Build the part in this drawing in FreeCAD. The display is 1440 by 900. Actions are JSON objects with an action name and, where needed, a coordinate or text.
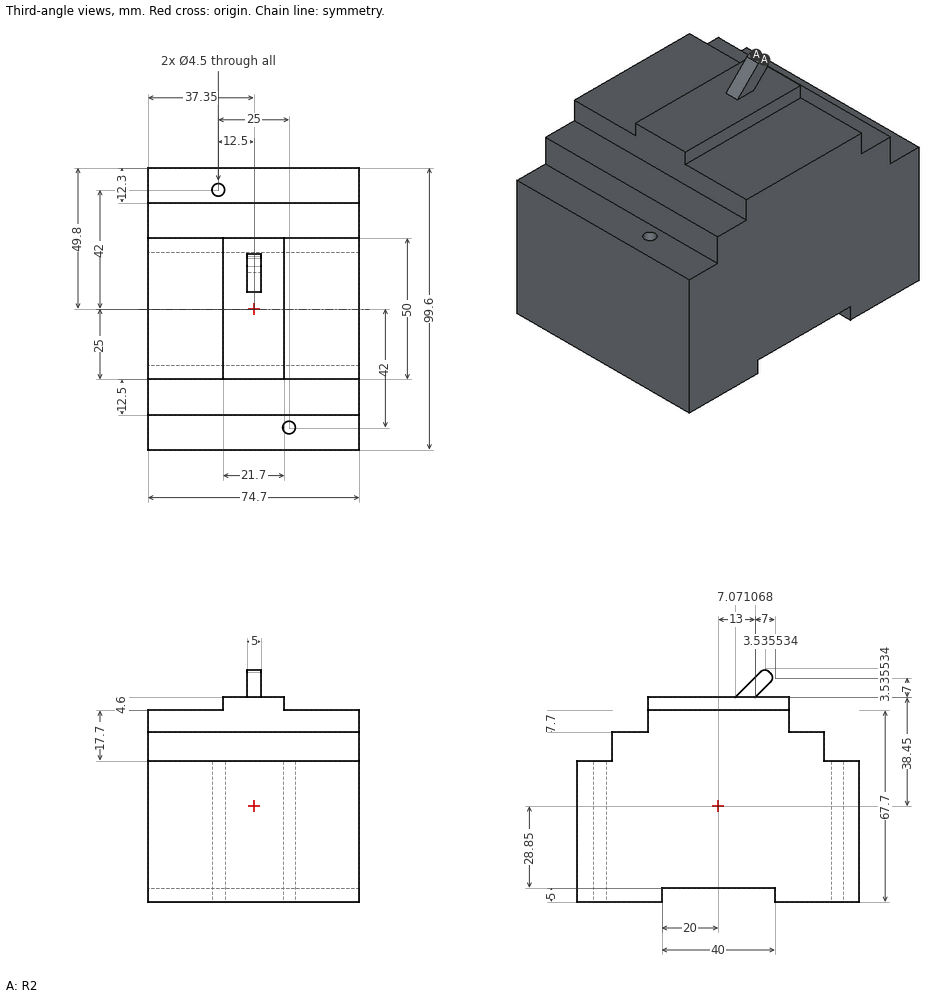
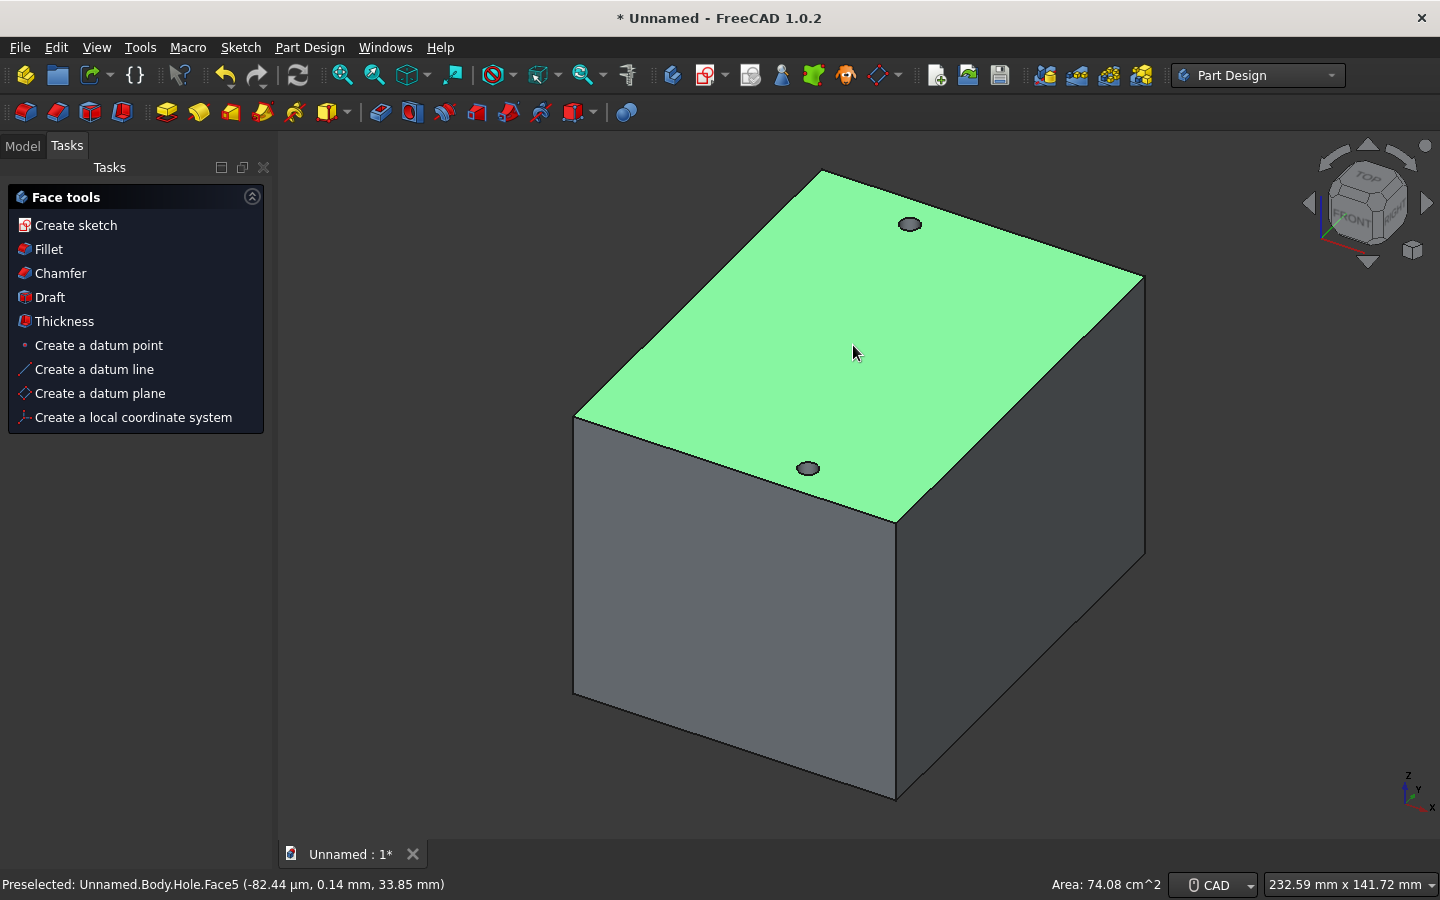
{"action": "left_click", "coordinate": [706, 76]}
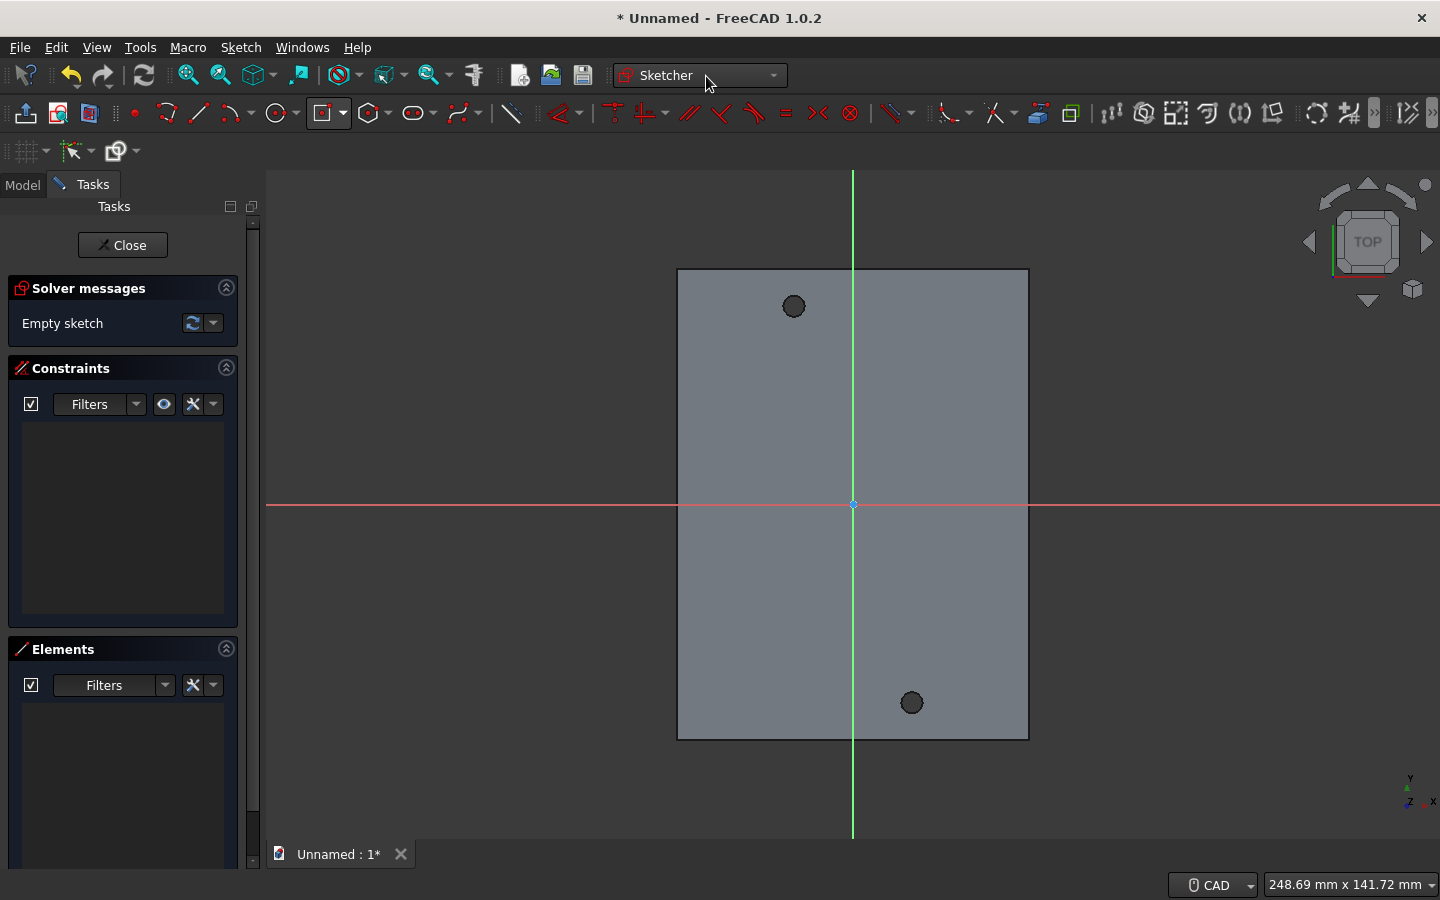
{"action": "left_click", "coordinate": [346, 114]}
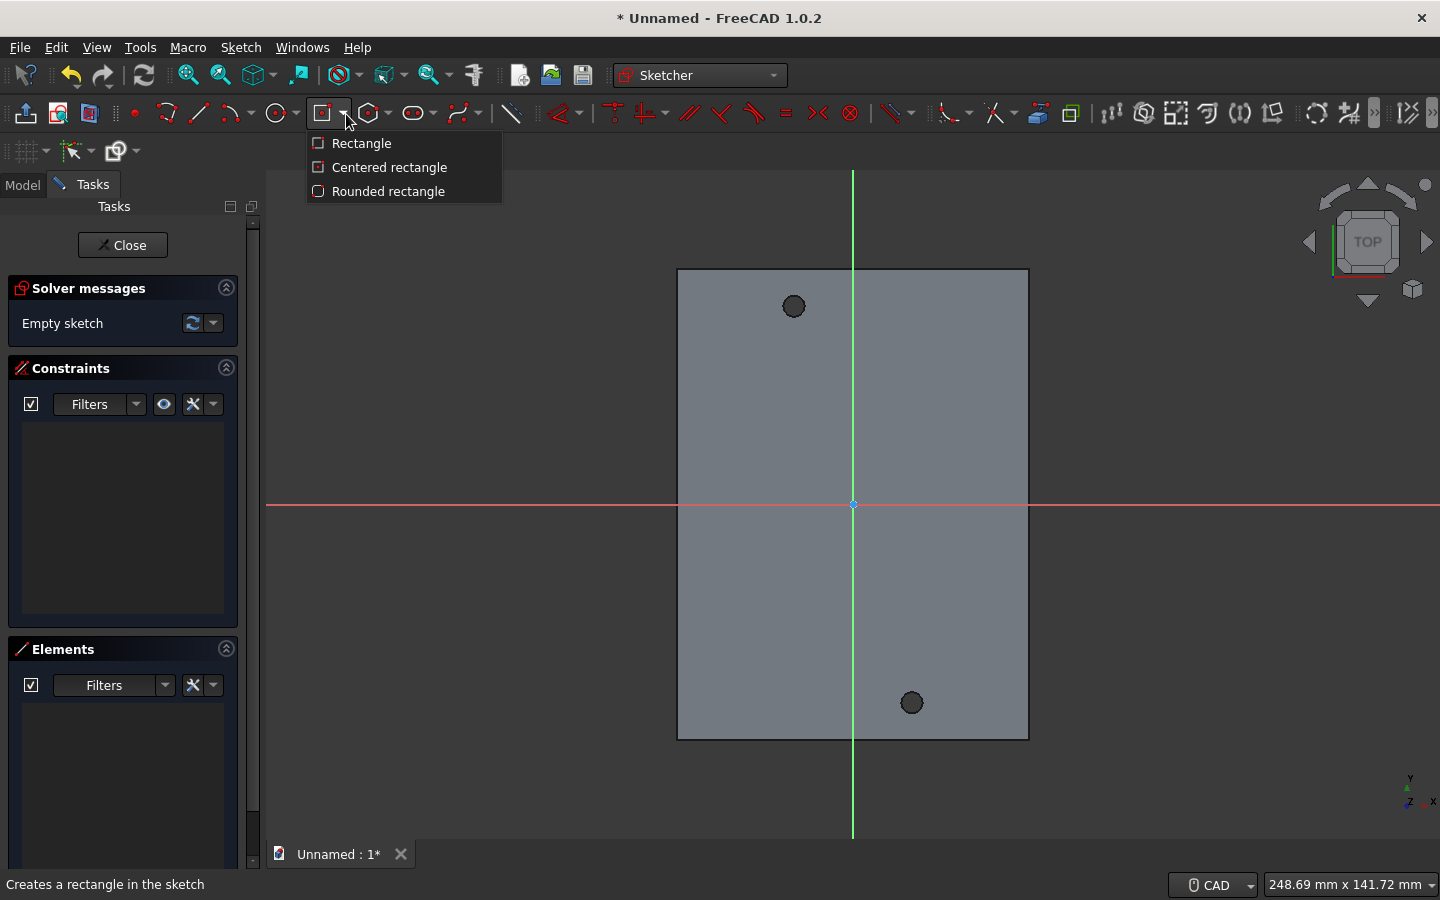
{"action": "left_click", "coordinate": [404, 143]}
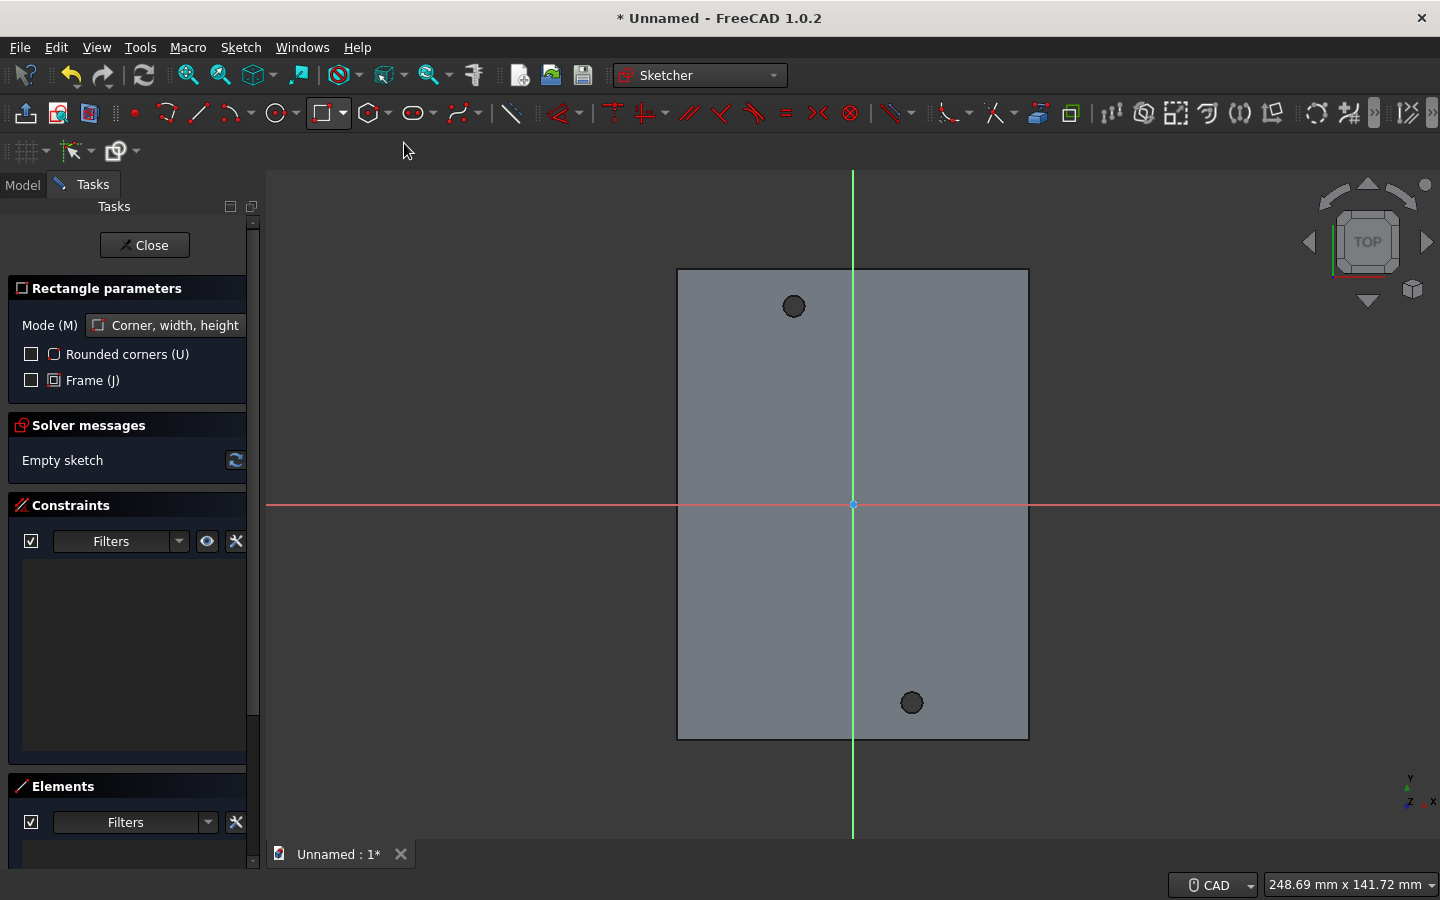
{"action": "left_click", "coordinate": [677, 269]}
{"action": "left_click", "coordinate": [1029, 327]}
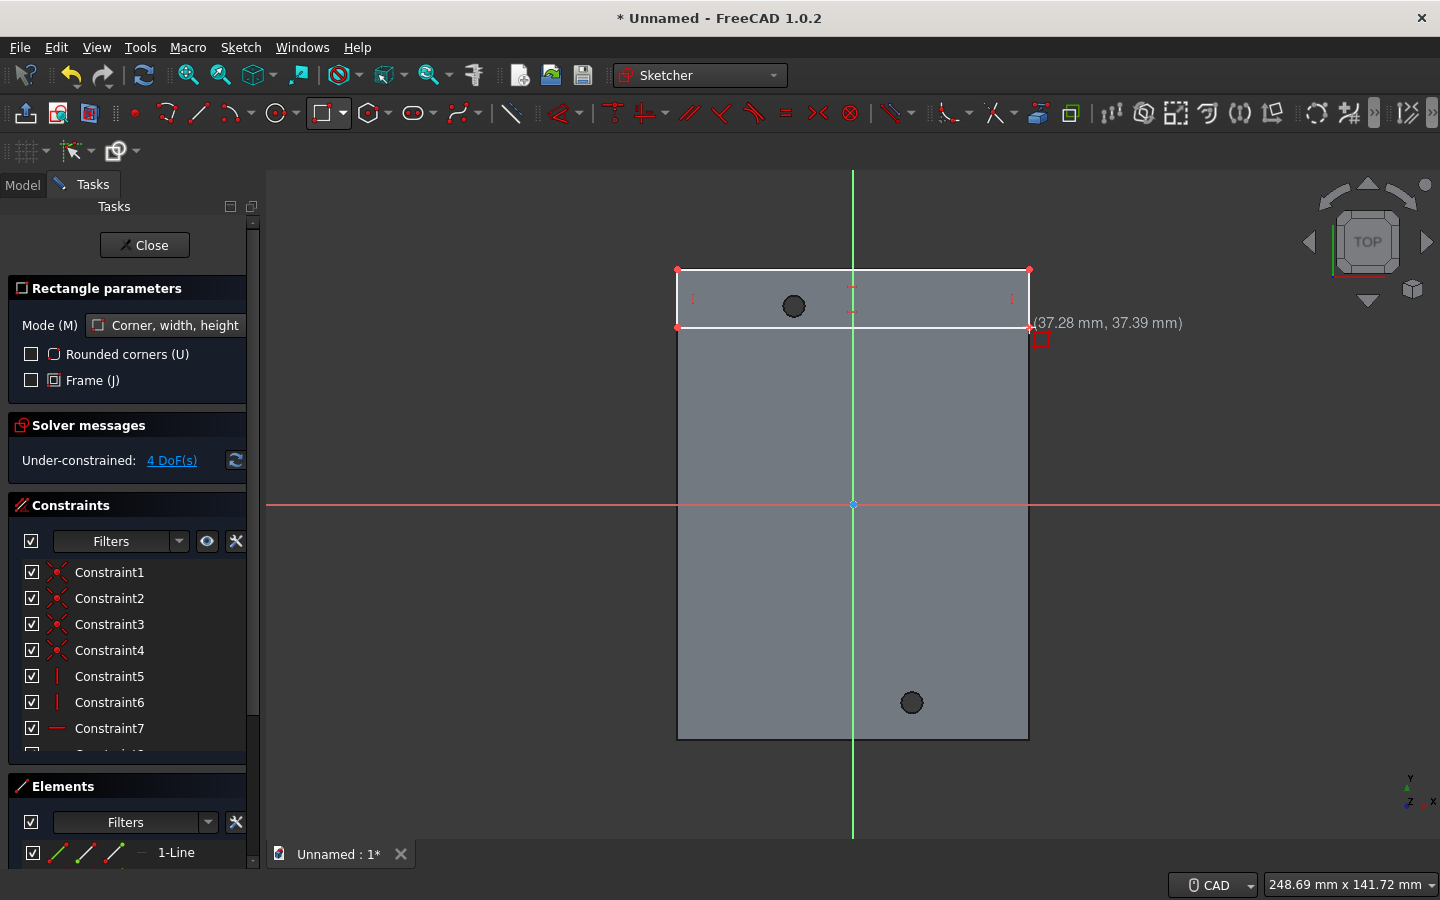
{"action": "left_click", "coordinate": [677, 682]}
{"action": "left_click", "coordinate": [1029, 740]}
{"action": "key", "text": "Escape"}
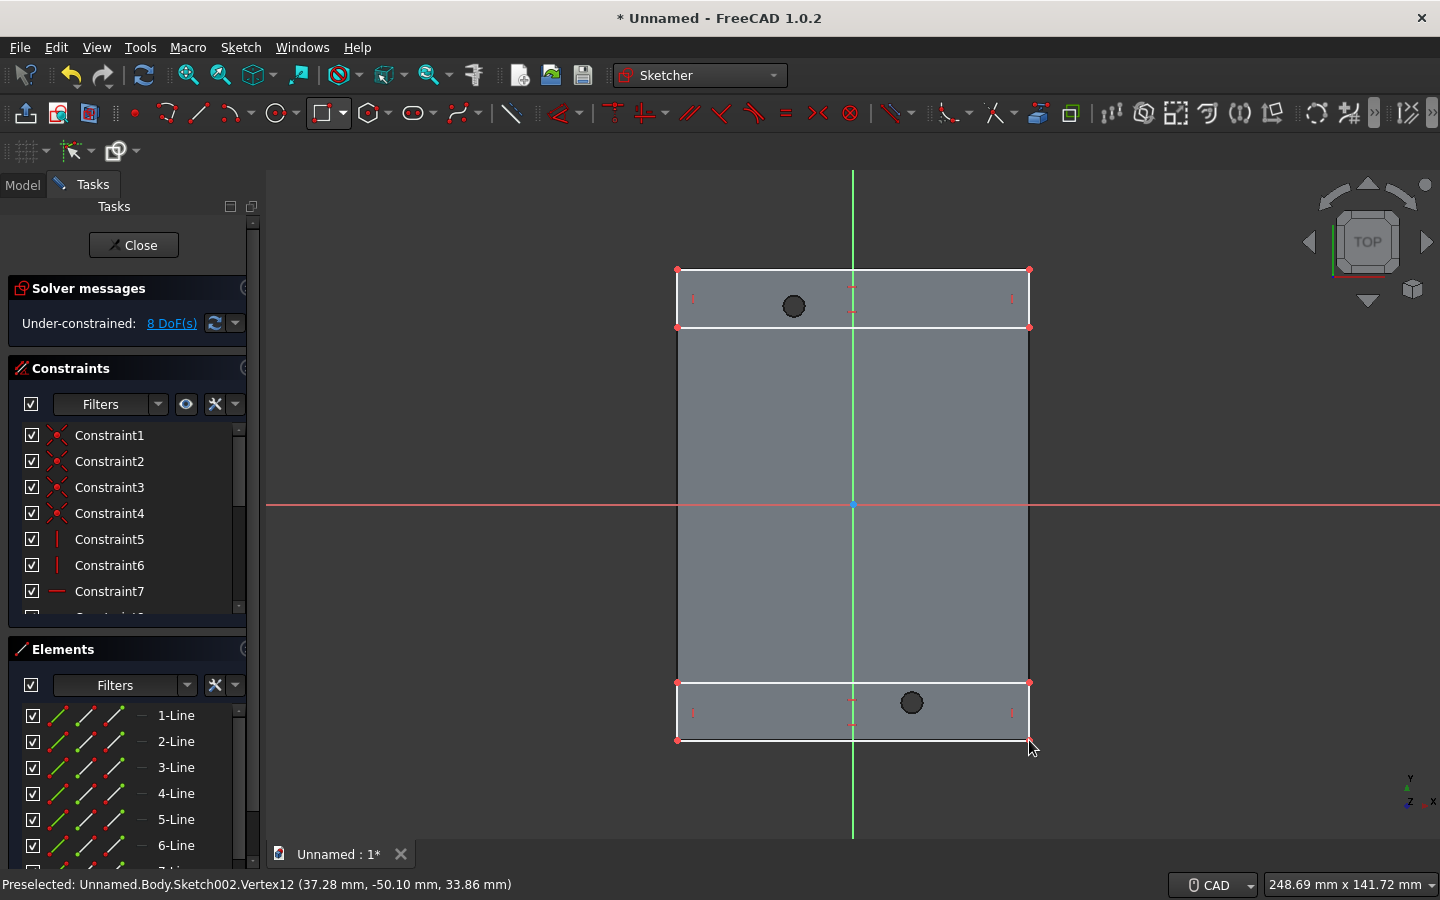
{"action": "left_click", "coordinate": [677, 328]}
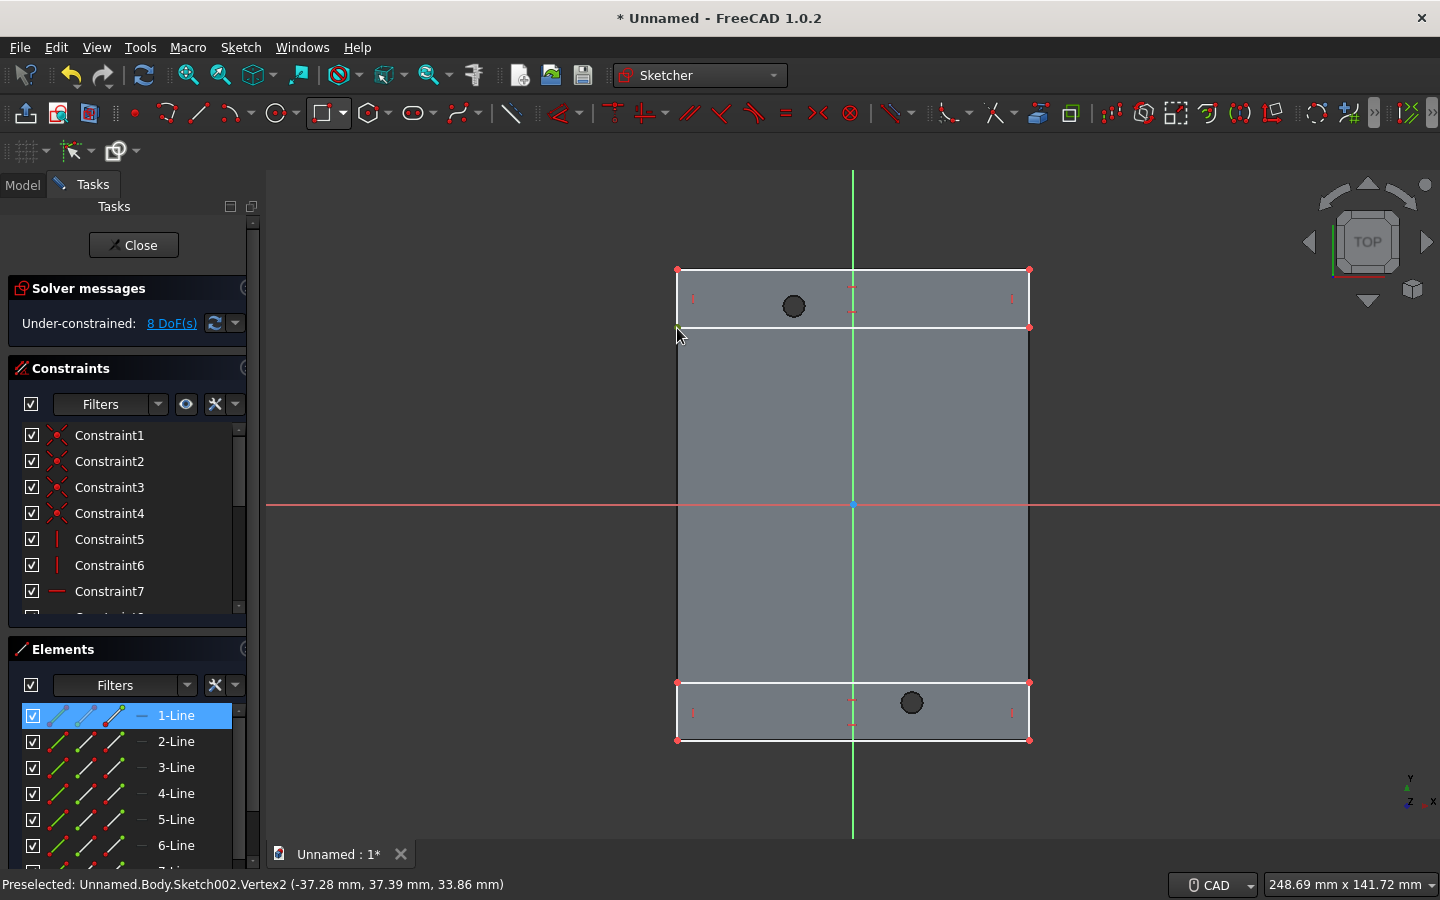
{"action": "left_click", "coordinate": [677, 683]}